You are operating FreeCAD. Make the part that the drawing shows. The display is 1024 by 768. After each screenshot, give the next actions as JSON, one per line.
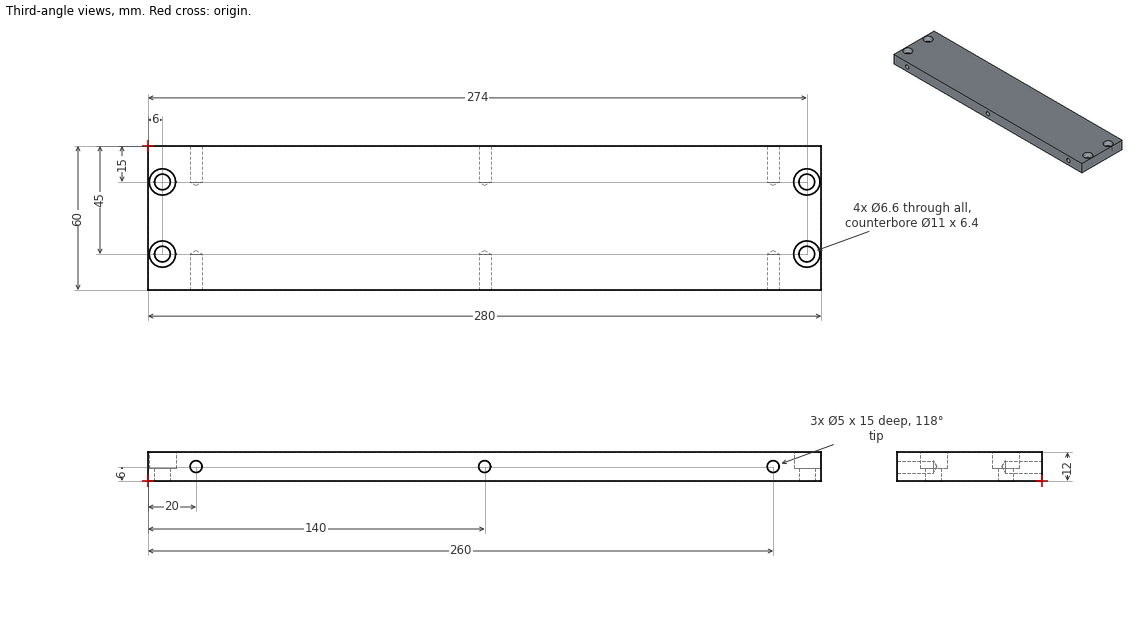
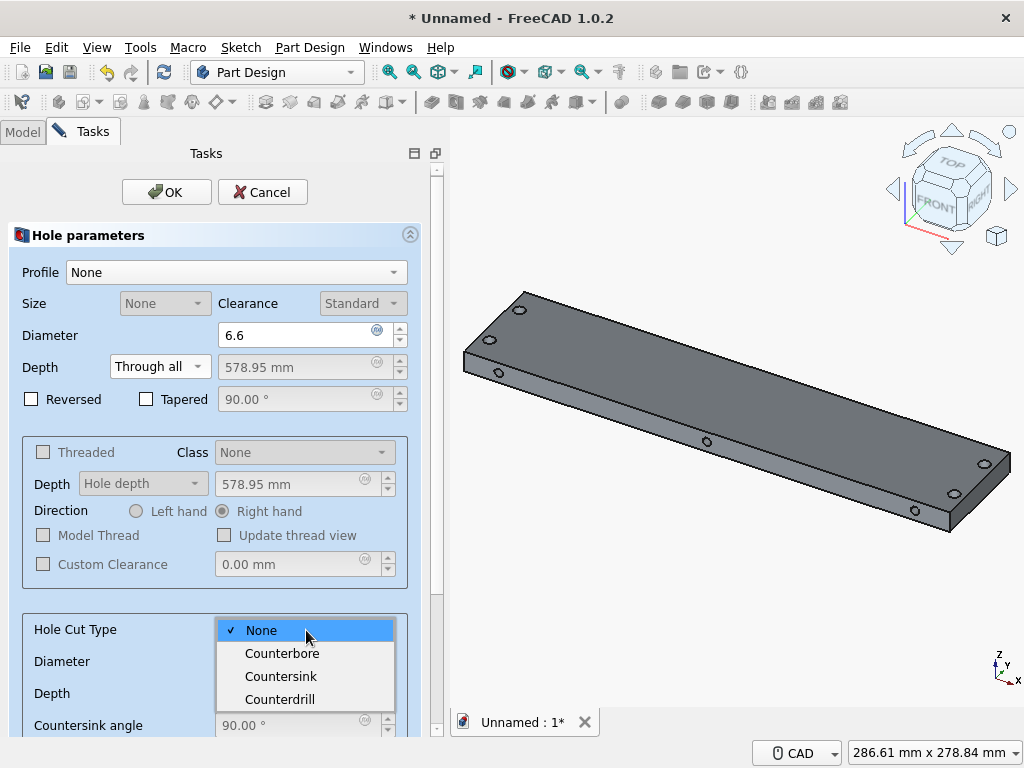
{"action": "left_click", "coordinate": [304, 654]}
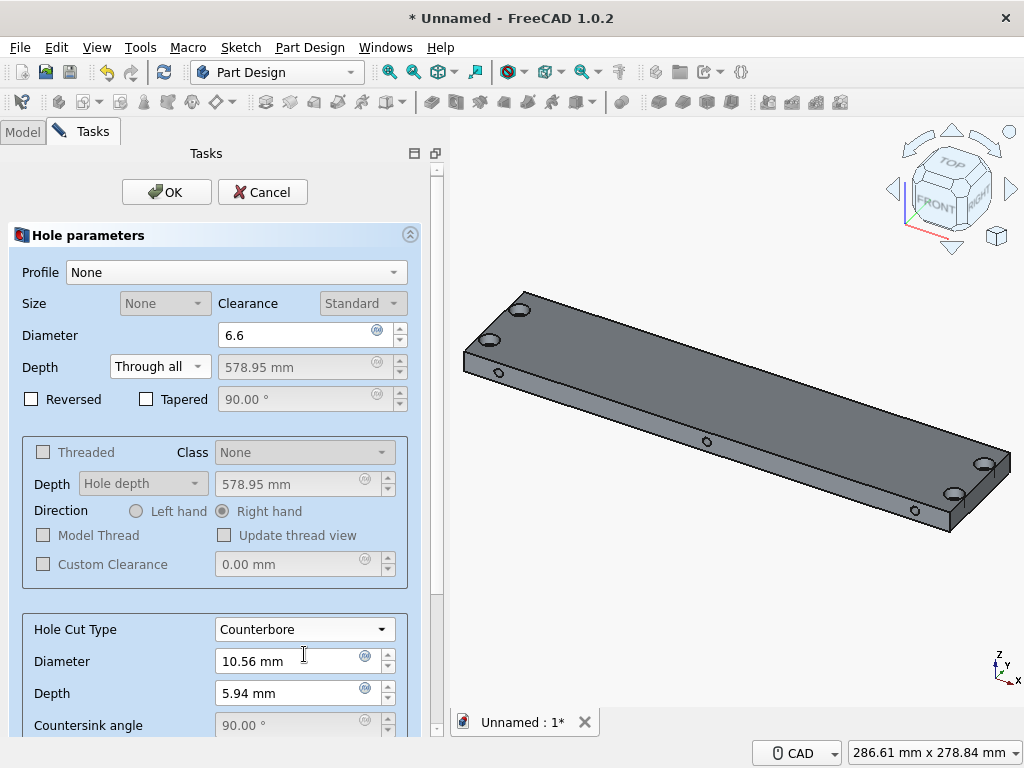
{"action": "triple_click", "coordinate": [298, 661]}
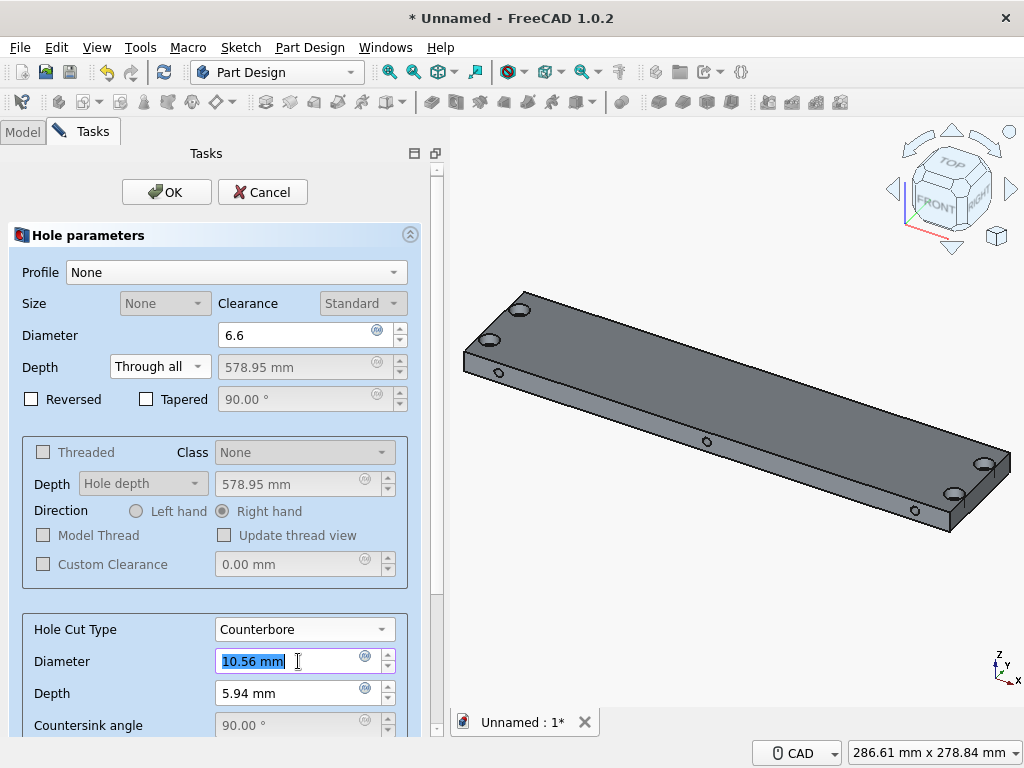
{"action": "type", "text": "11"}
{"action": "key", "text": "Tab"}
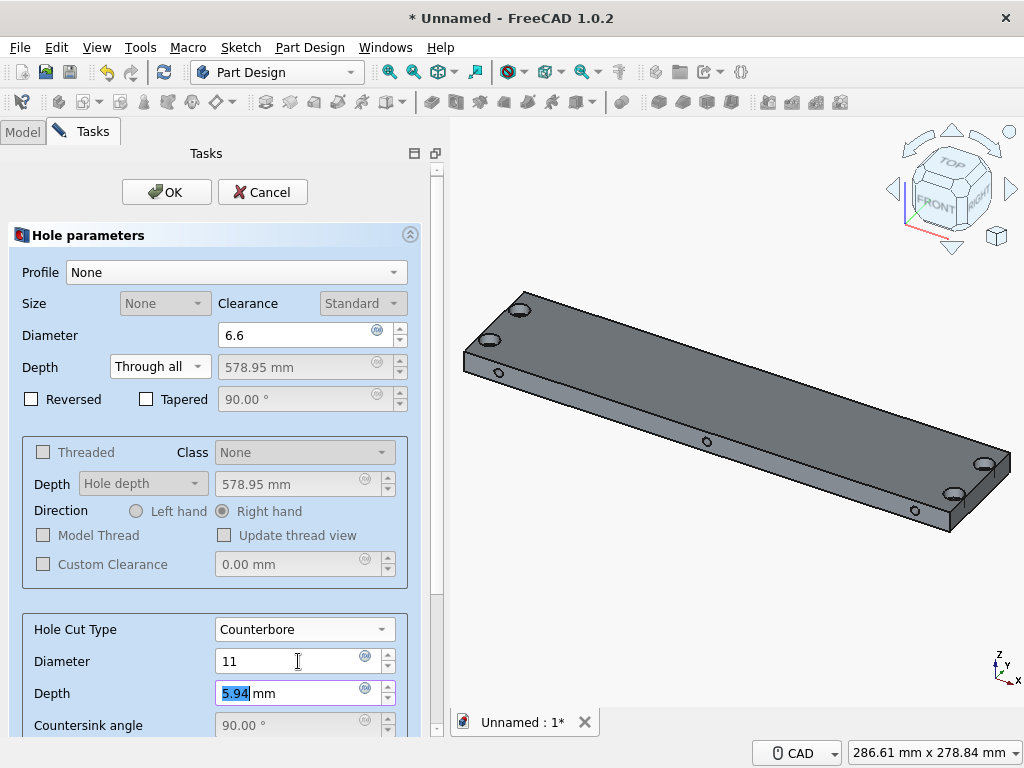
{"action": "type", "text": "6.4"}
{"action": "key", "text": "Tab"}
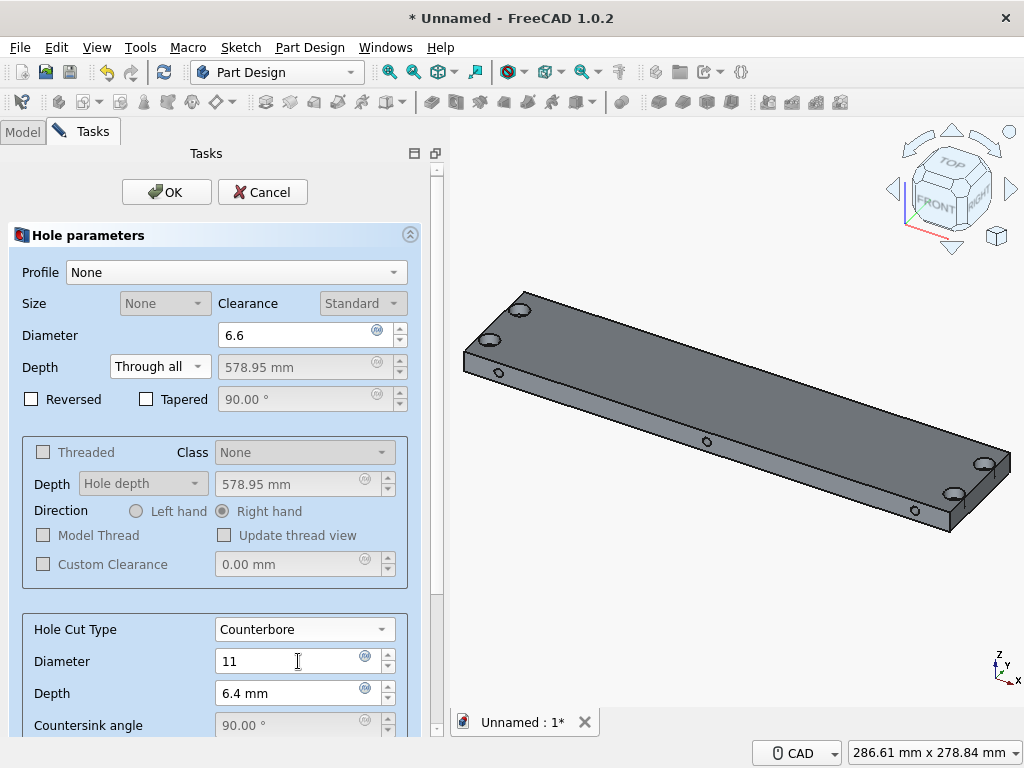
{"action": "left_click", "coordinate": [167, 192]}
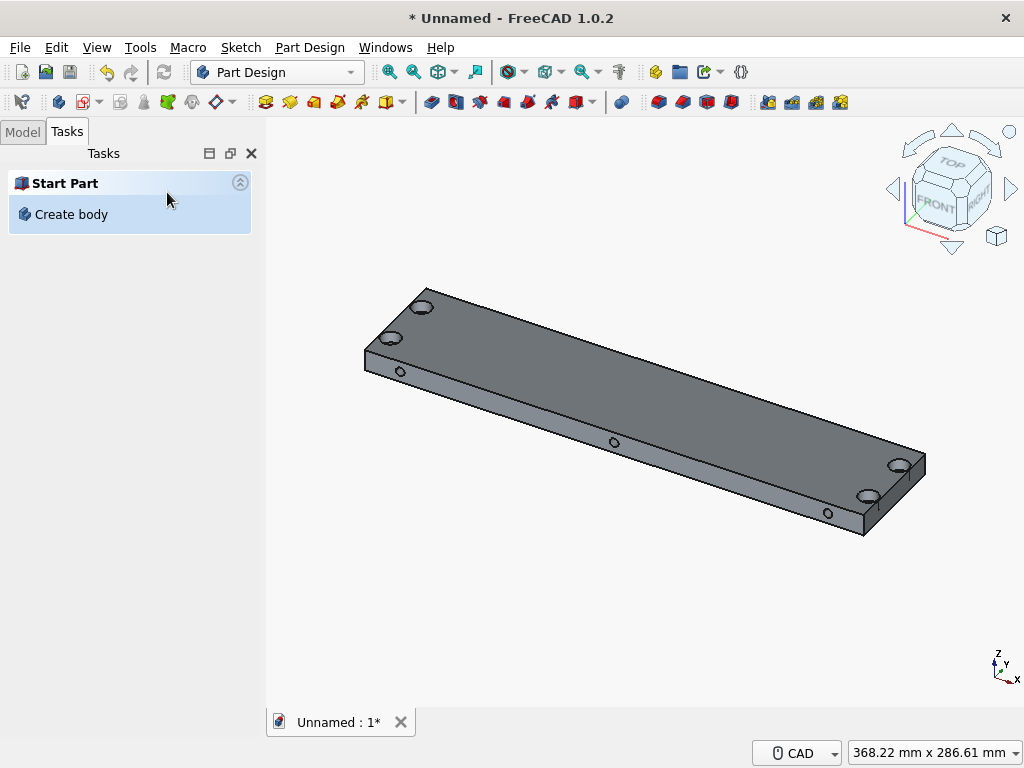
{"action": "key", "text": "0"}